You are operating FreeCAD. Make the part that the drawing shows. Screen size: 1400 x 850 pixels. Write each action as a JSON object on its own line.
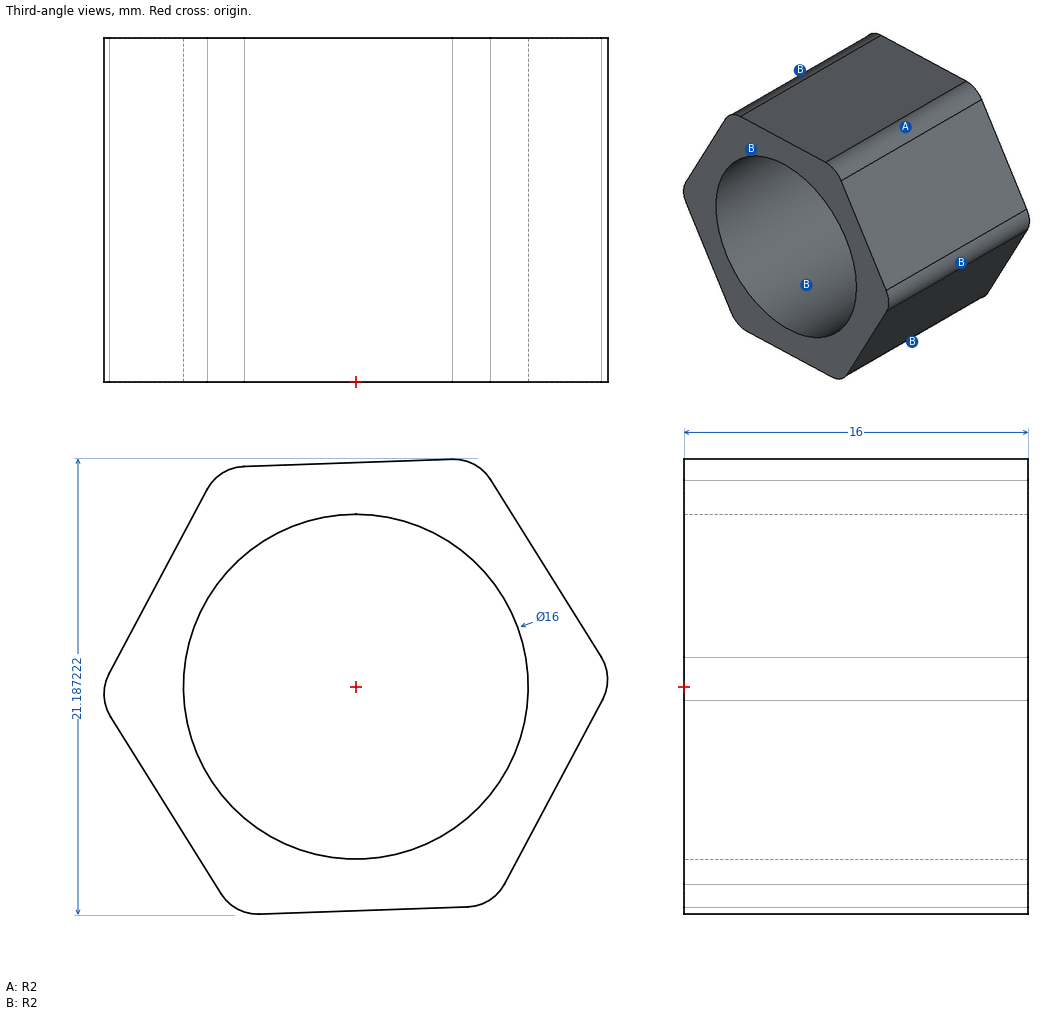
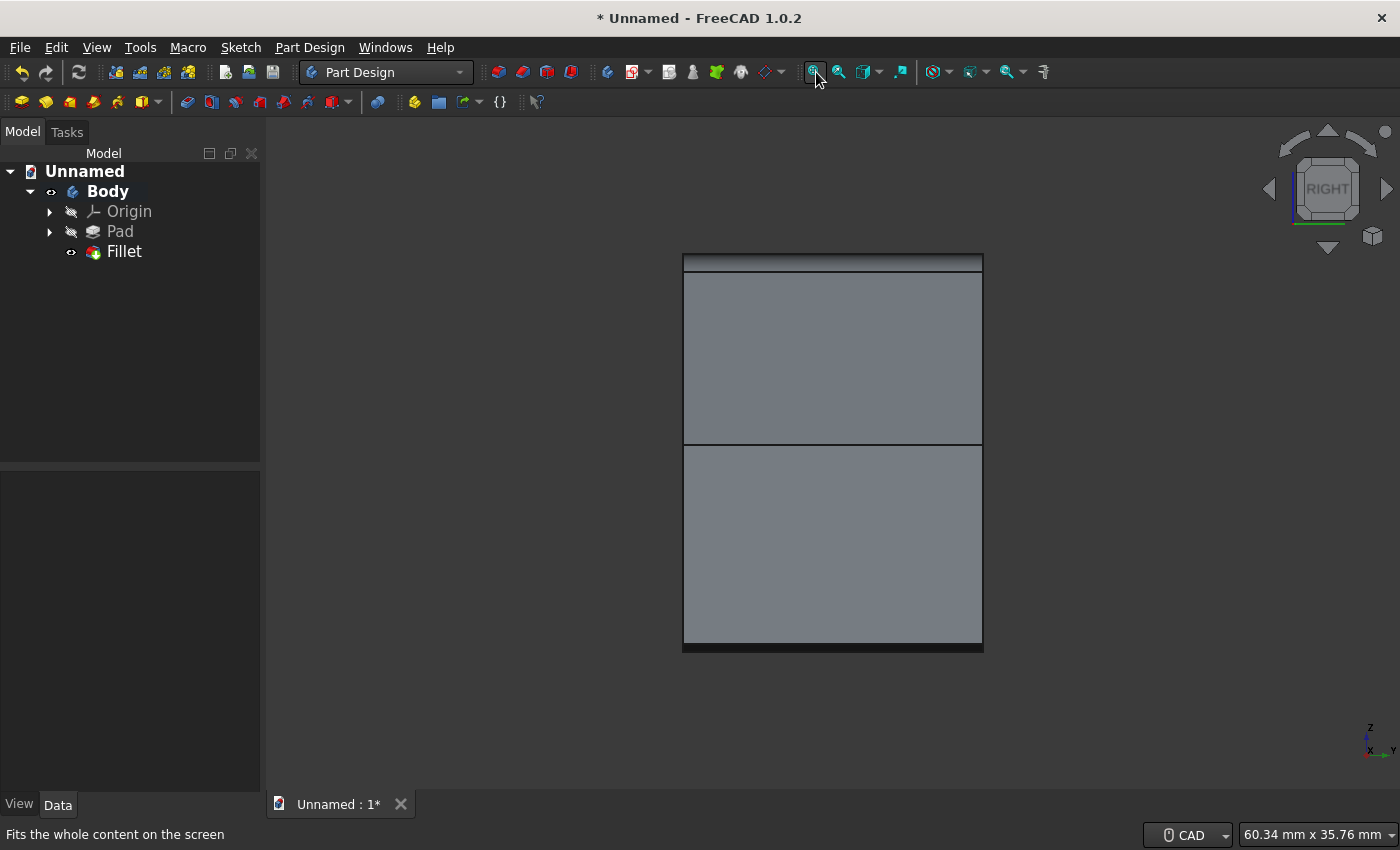
{"action": "left_click", "coordinate": [833, 444]}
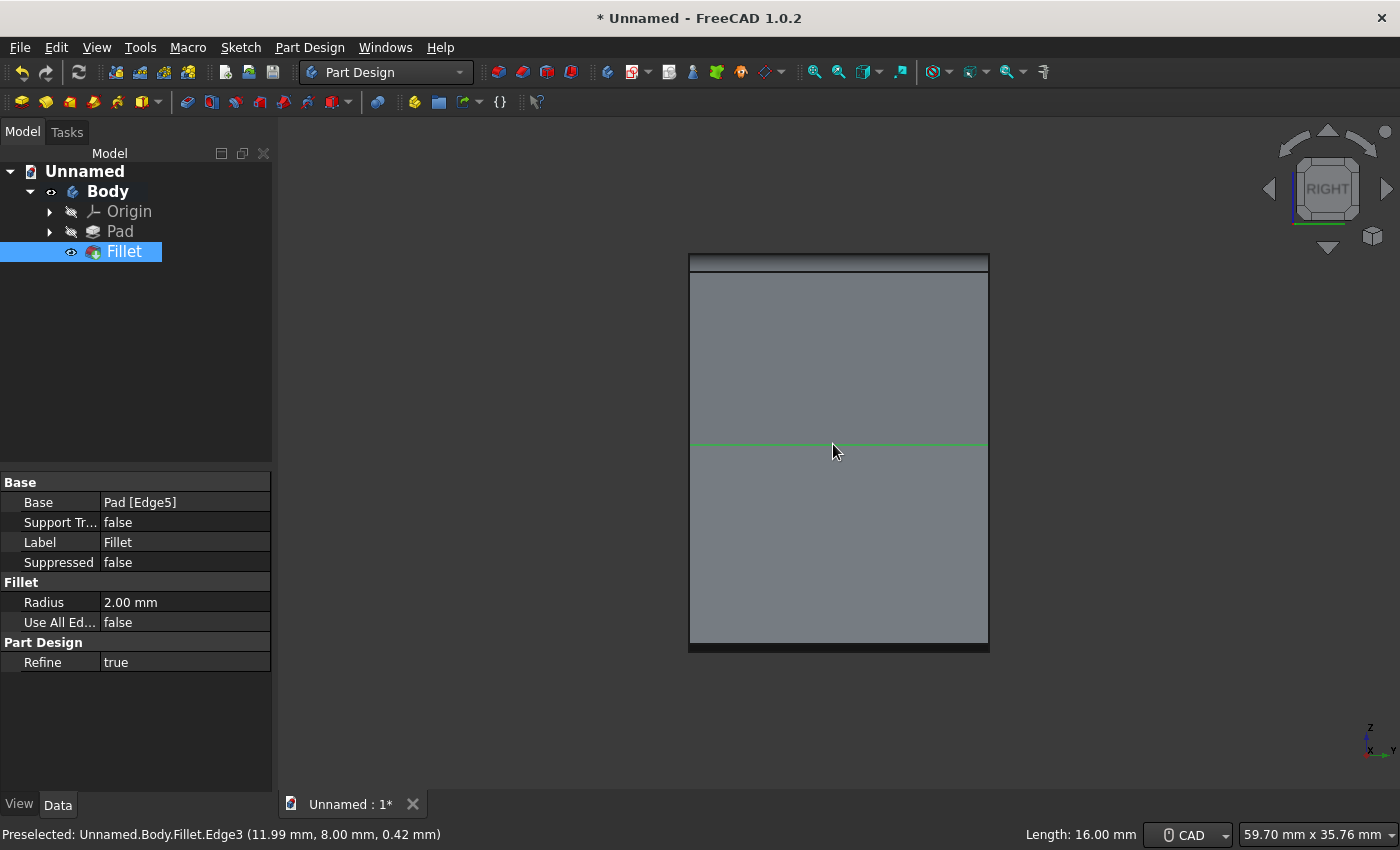
{"action": "key", "text": "5"}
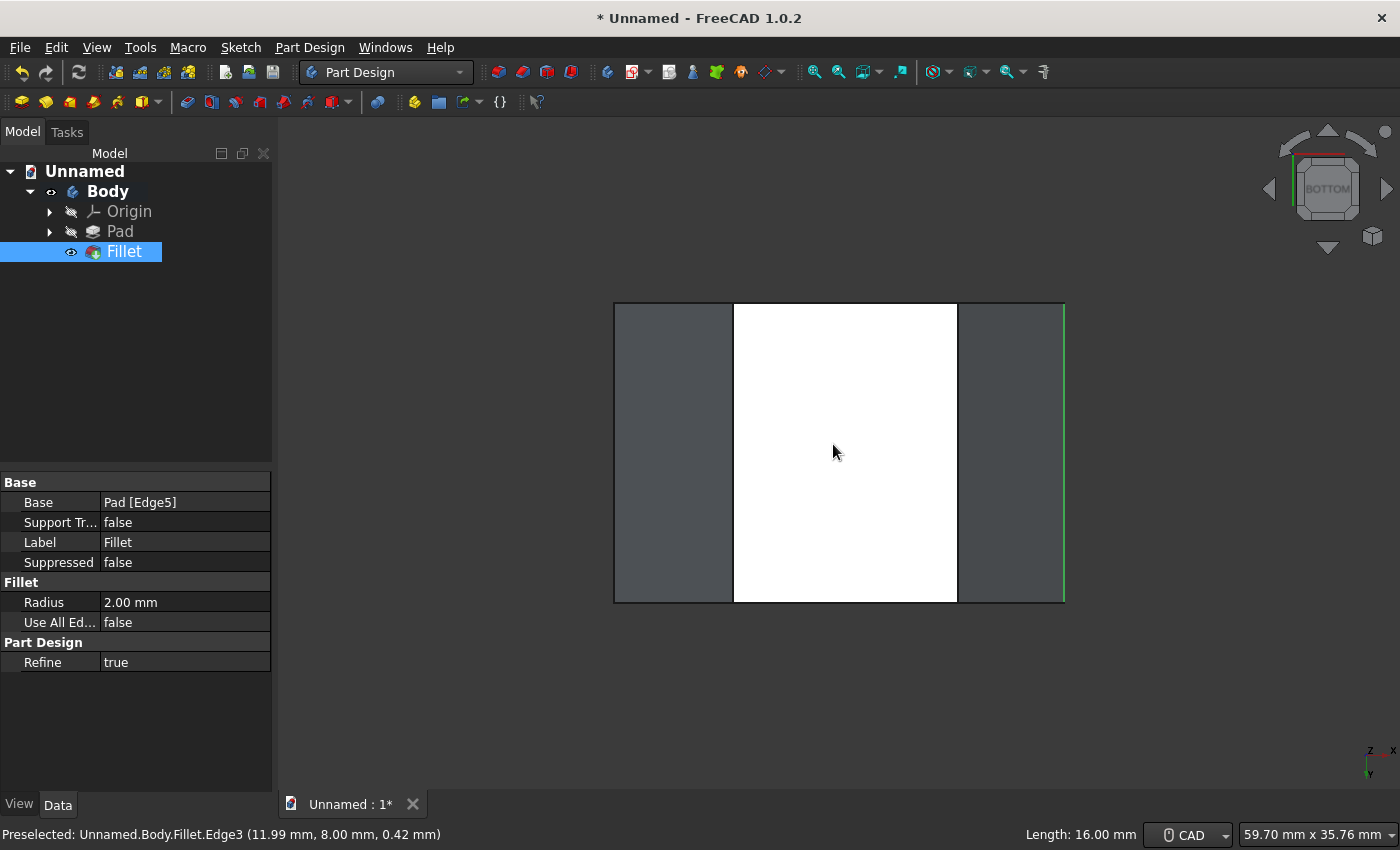
{"action": "left_click", "coordinate": [816, 72]}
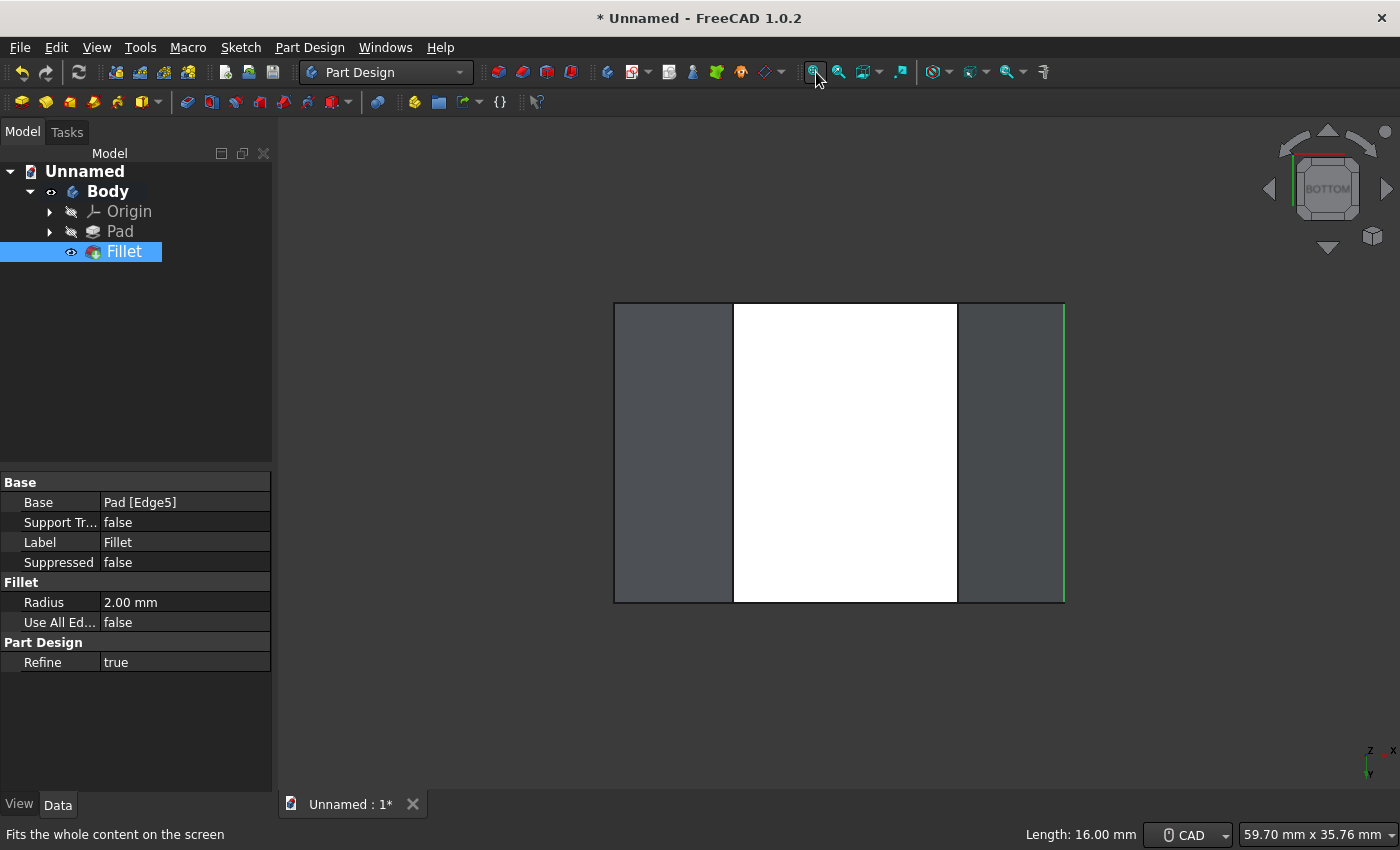
{"action": "left_click", "coordinate": [733, 452], "text": "ctrl"}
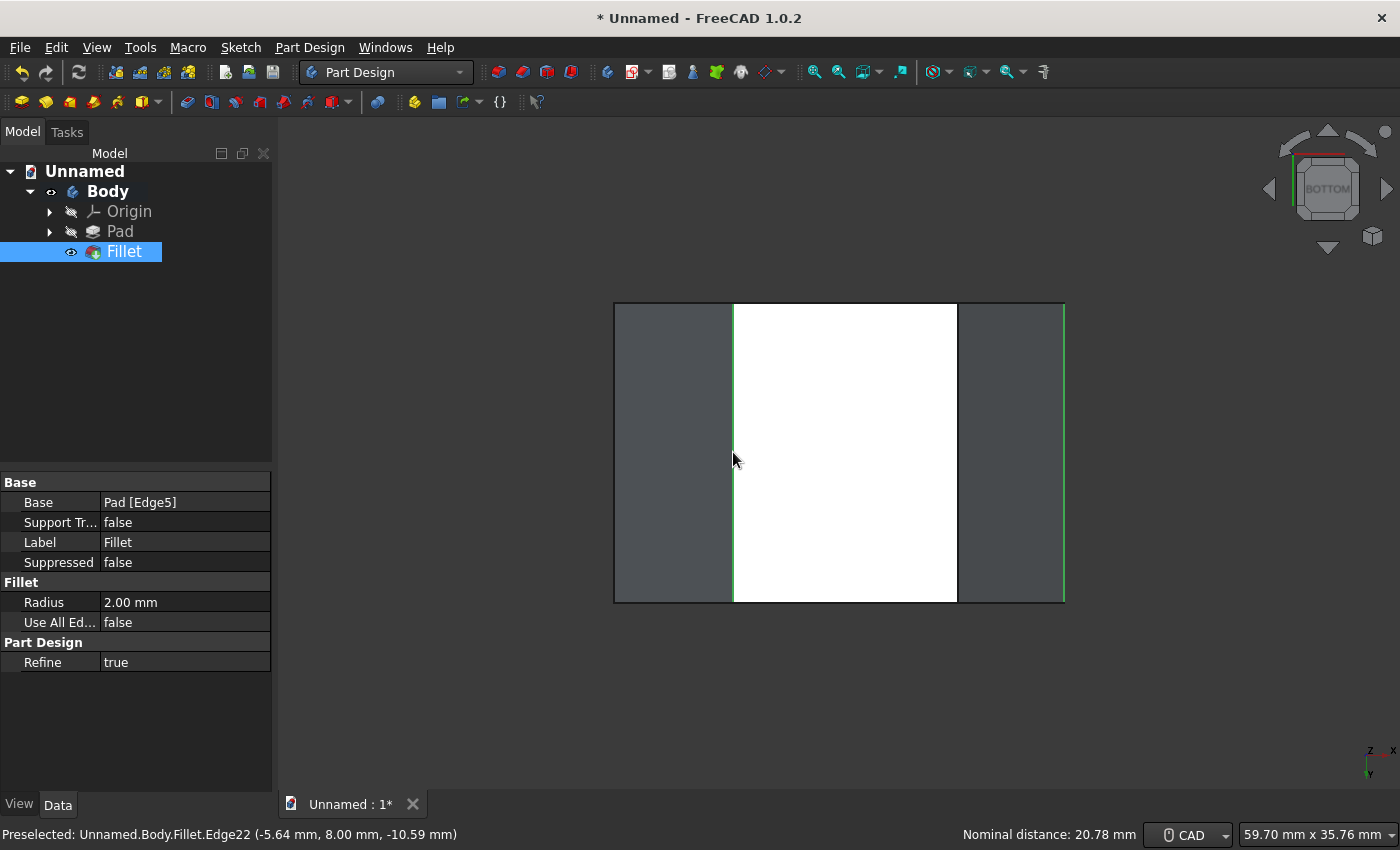
{"action": "key", "text": "4"}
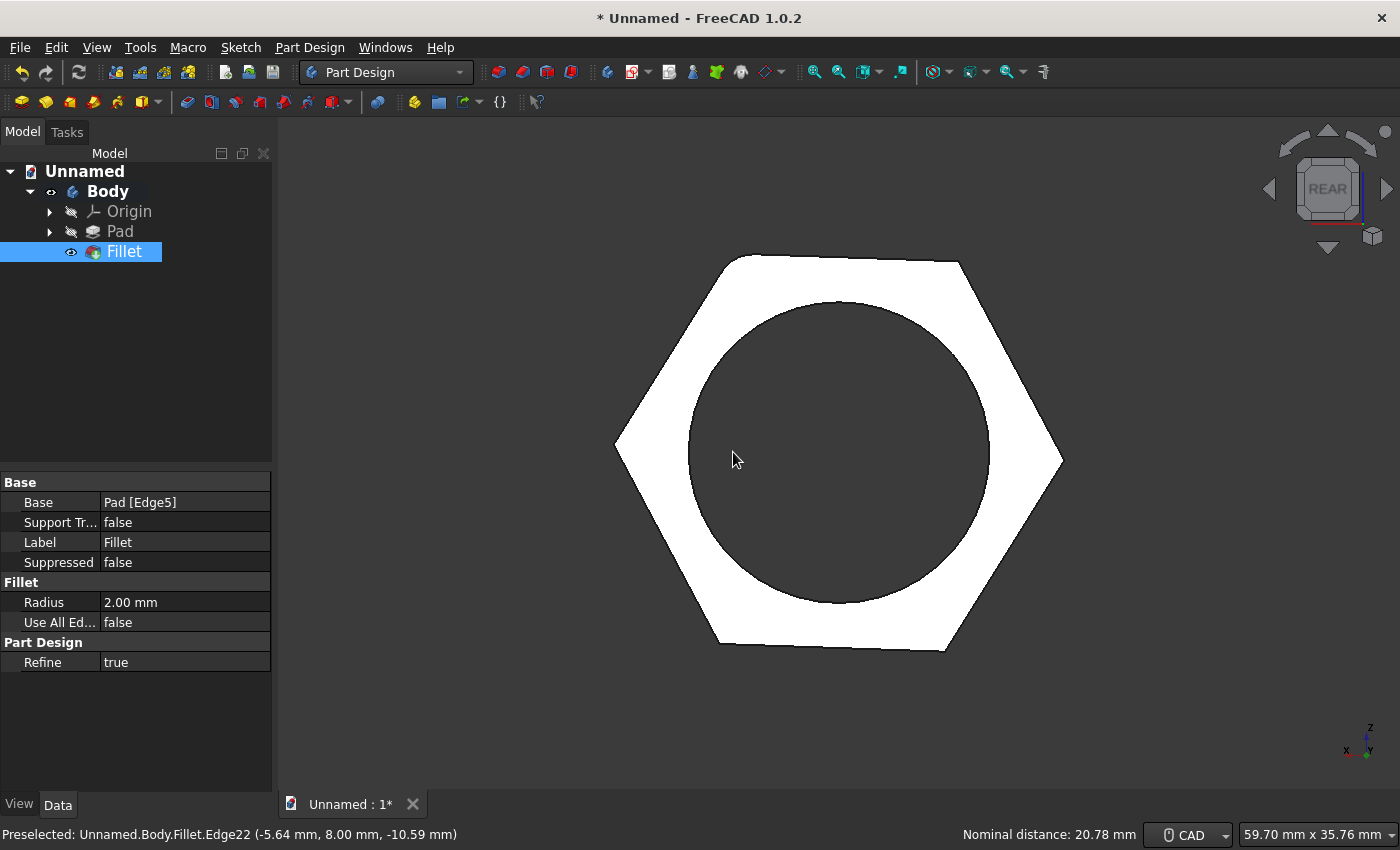
{"action": "key", "text": "6"}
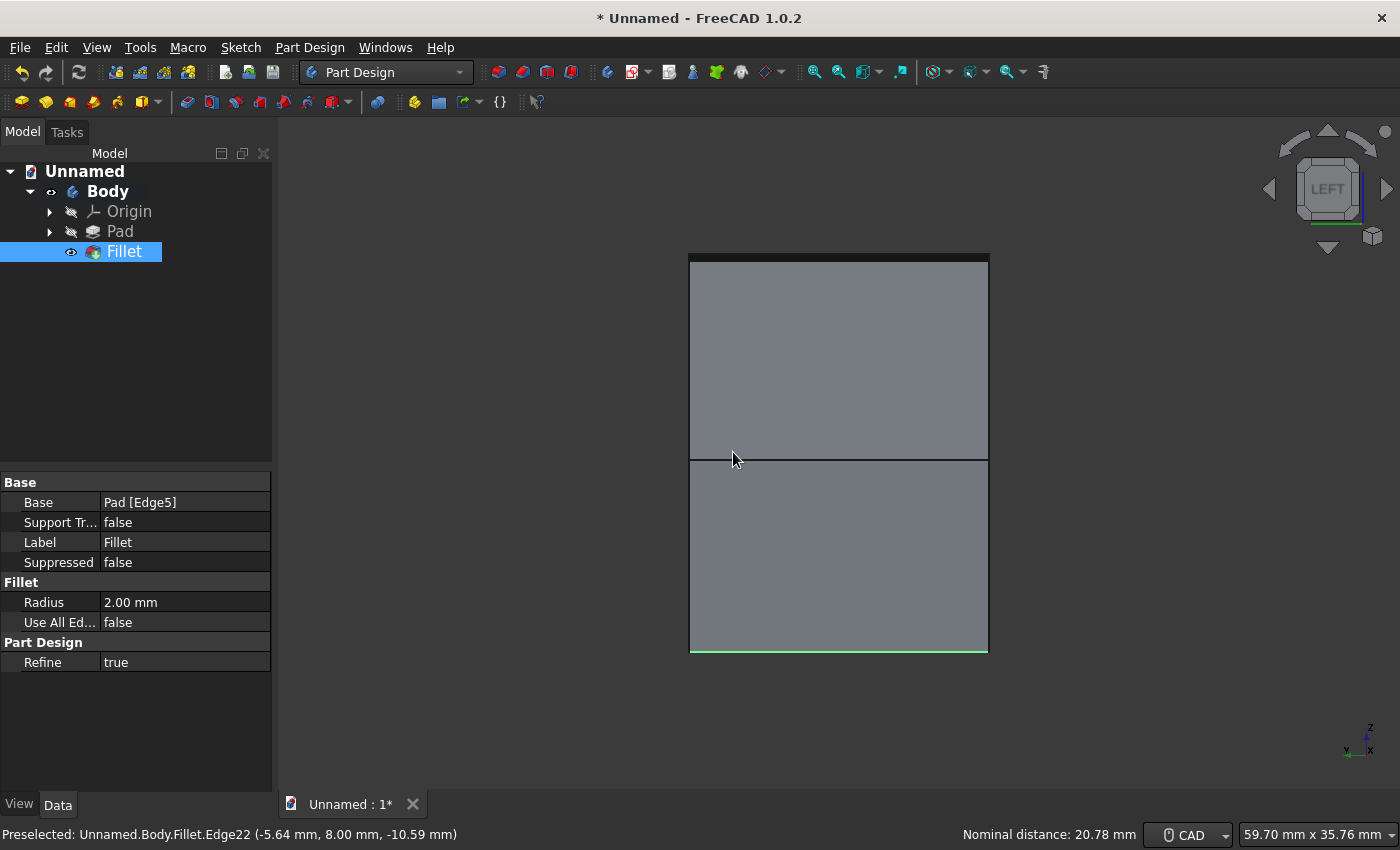
{"action": "left_click", "coordinate": [839, 459], "text": "ctrl"}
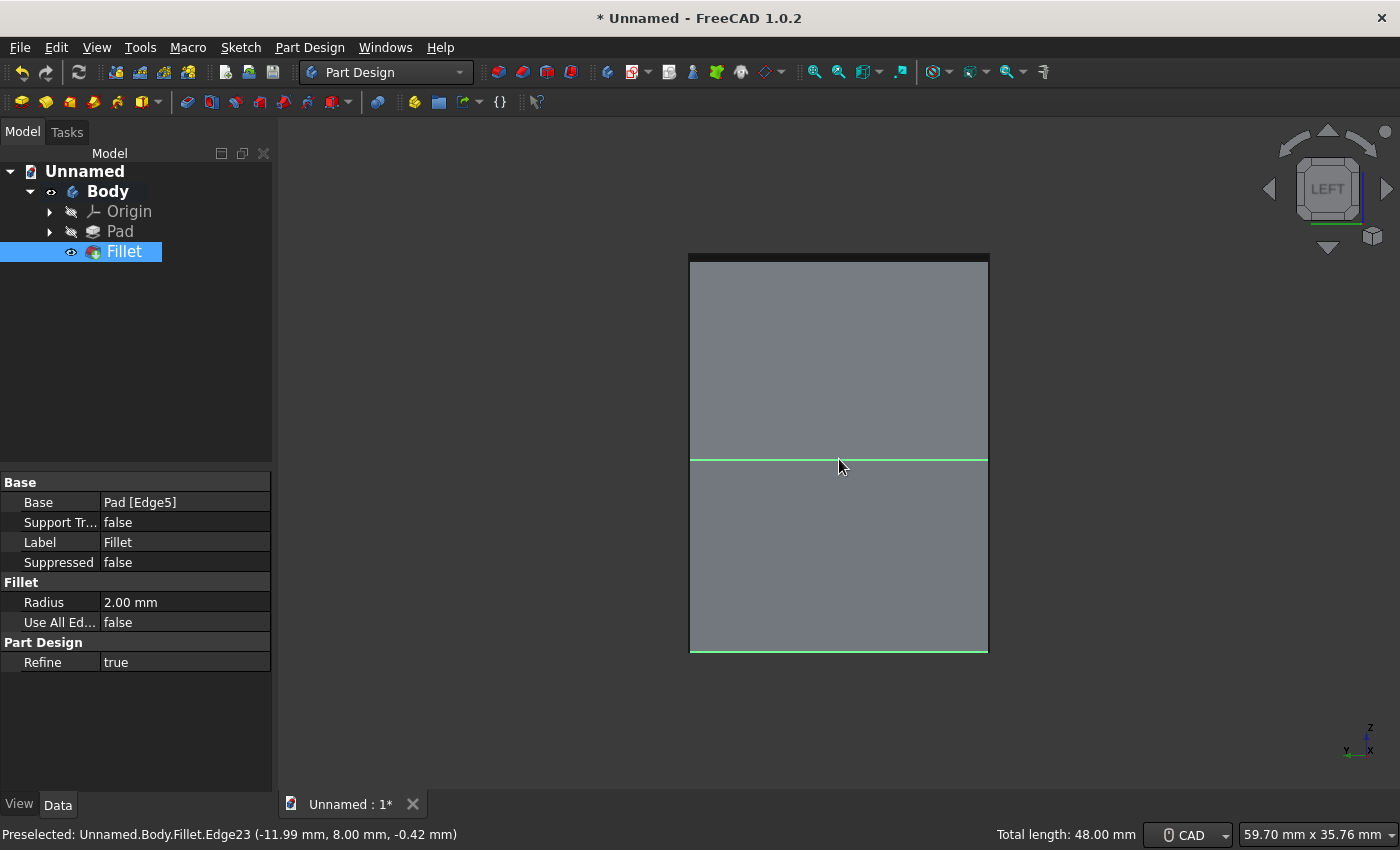
{"action": "key", "text": "v 3"}